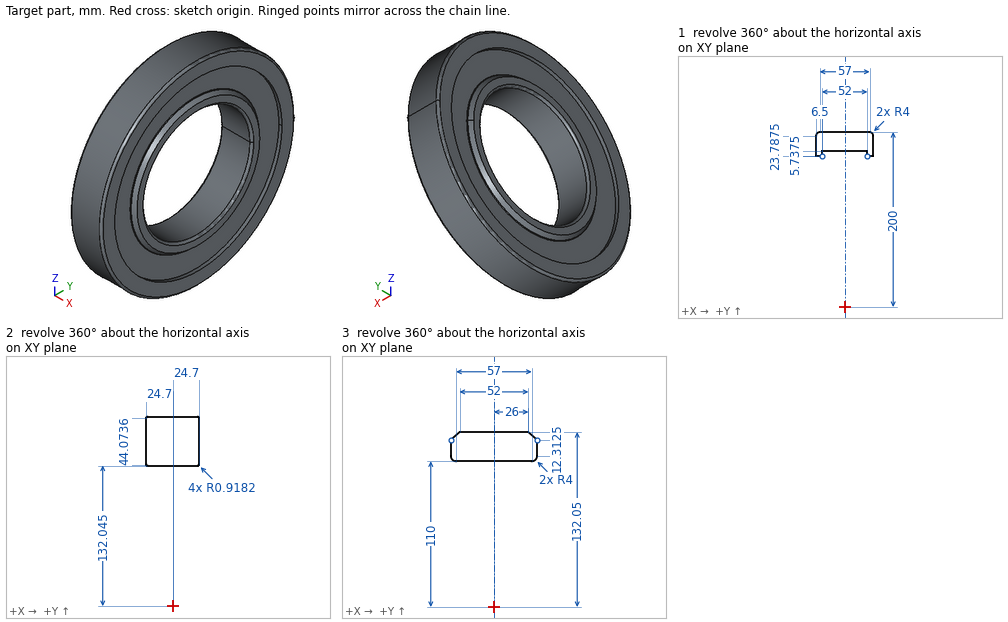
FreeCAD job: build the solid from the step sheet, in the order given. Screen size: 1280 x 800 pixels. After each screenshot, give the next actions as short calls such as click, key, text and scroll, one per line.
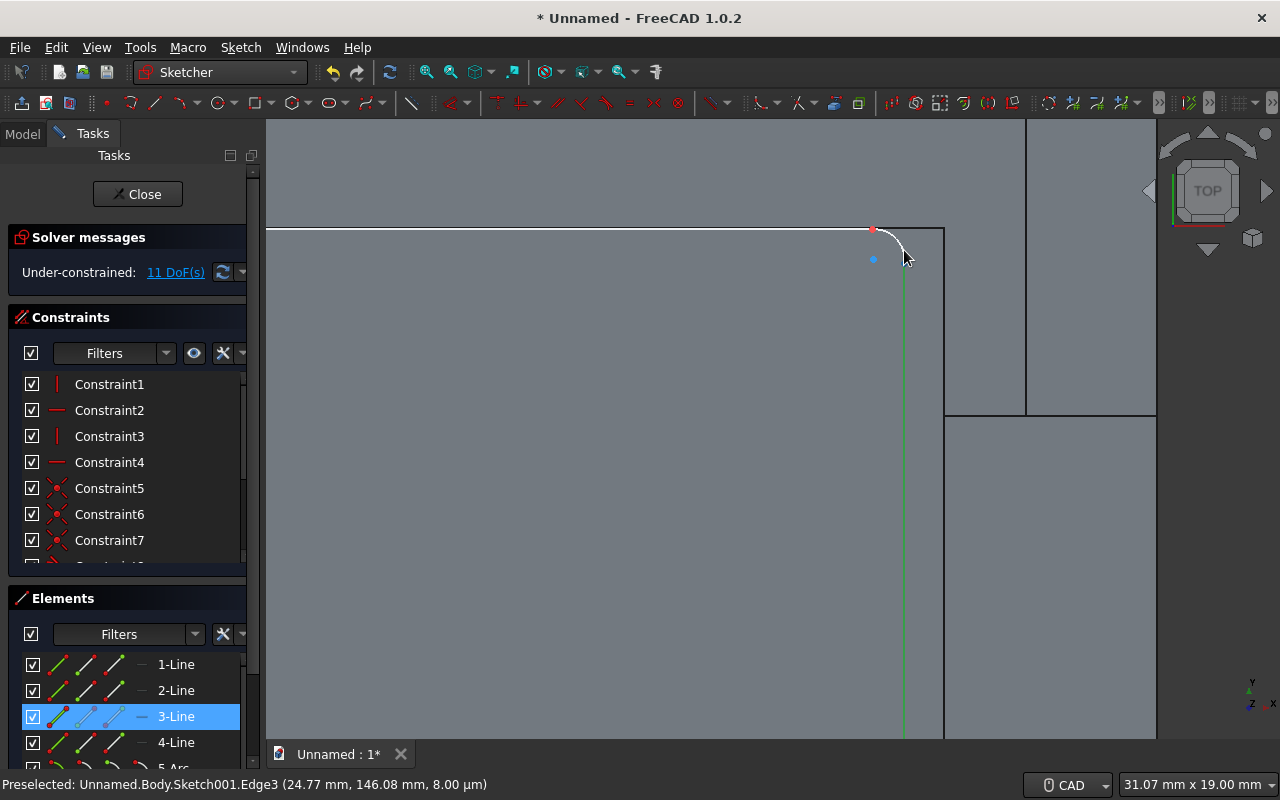
click(902, 248)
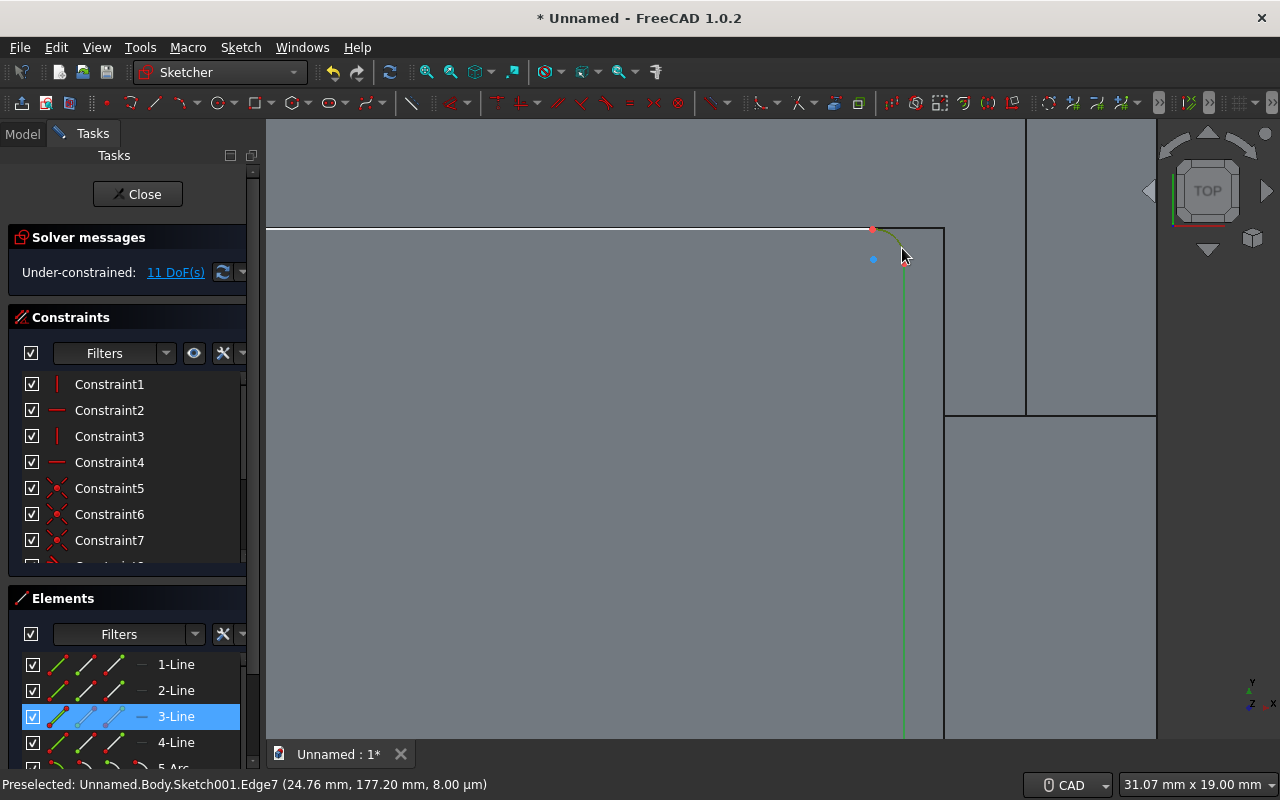
click(606, 104)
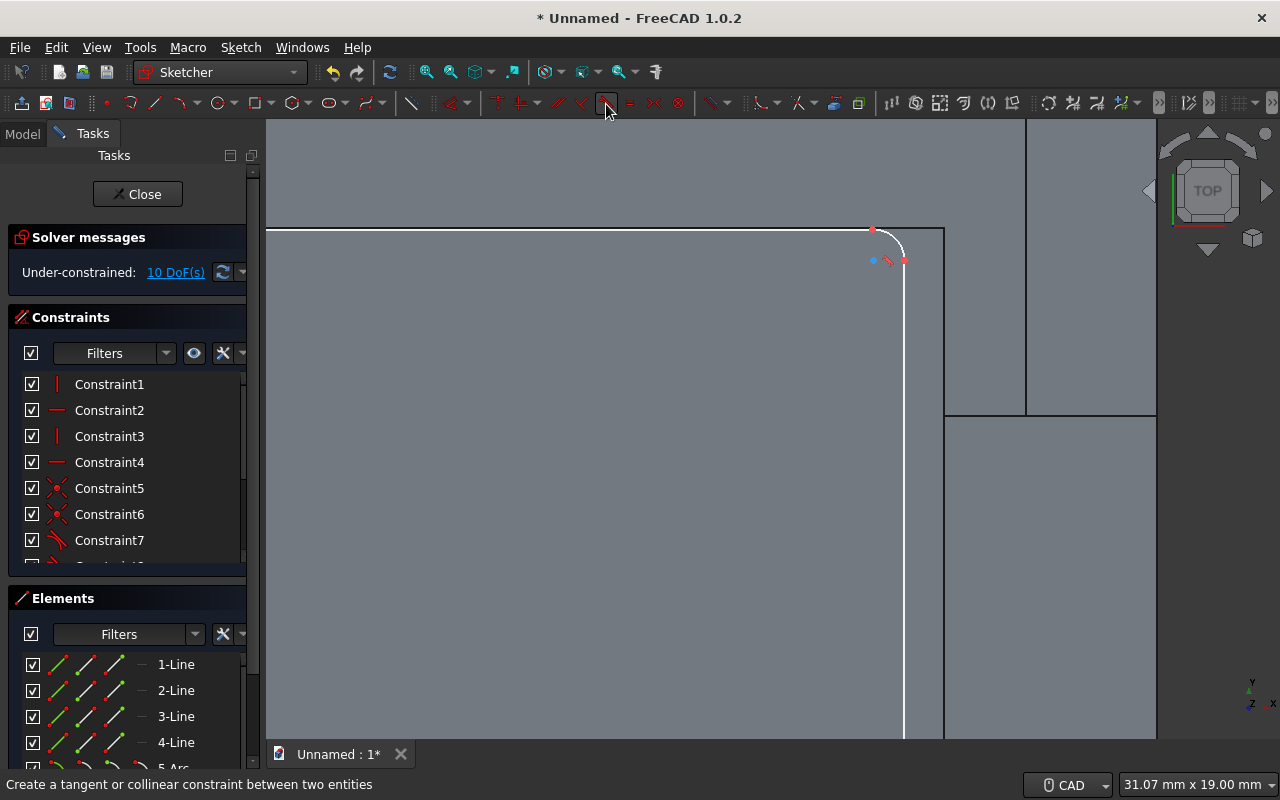
scroll(904, 250, down, 7)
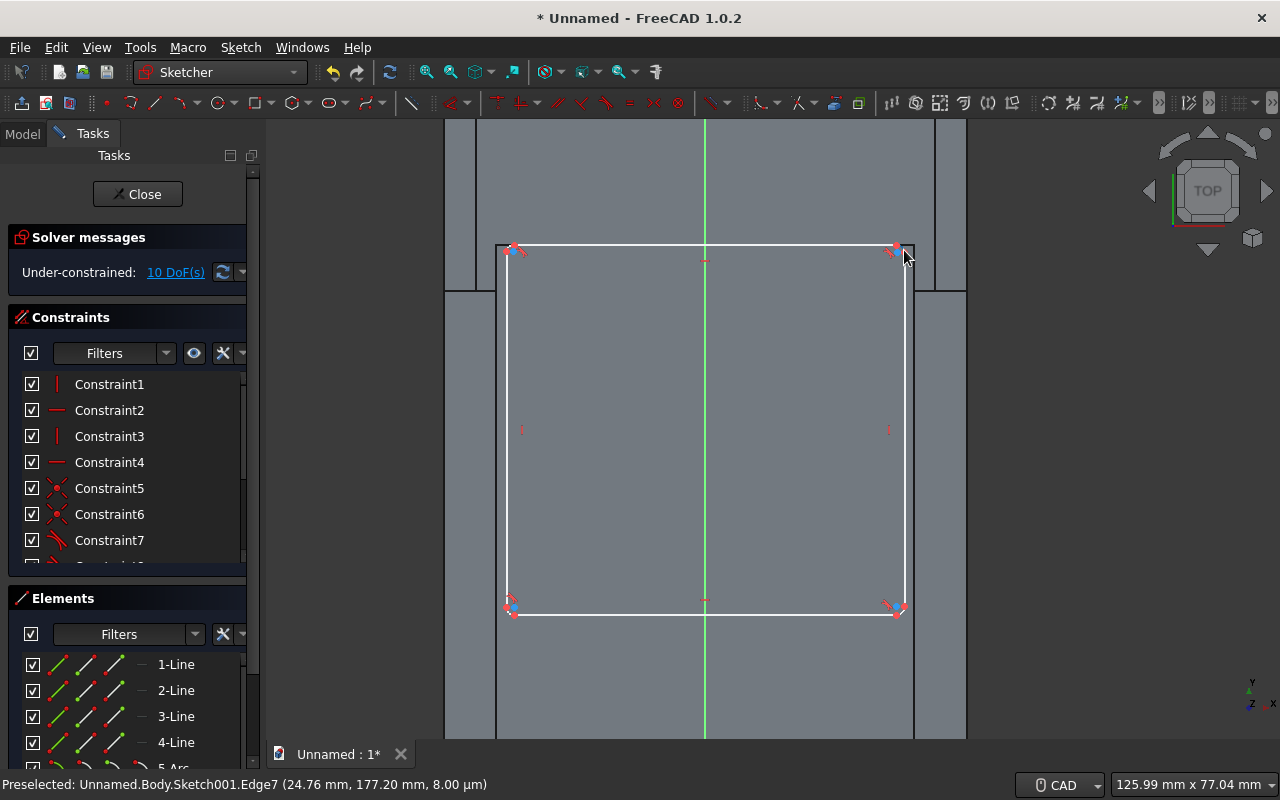
click(782, 245)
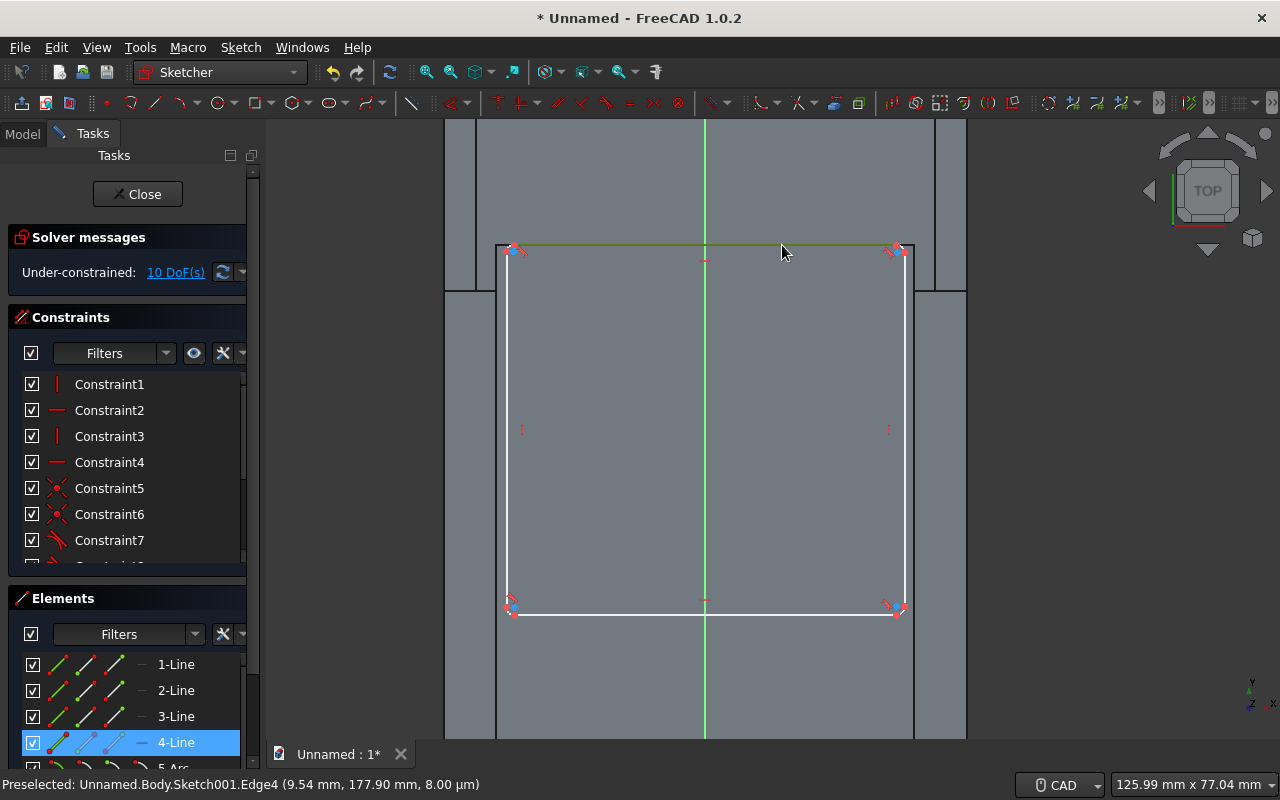
scroll(902, 247, up, 5)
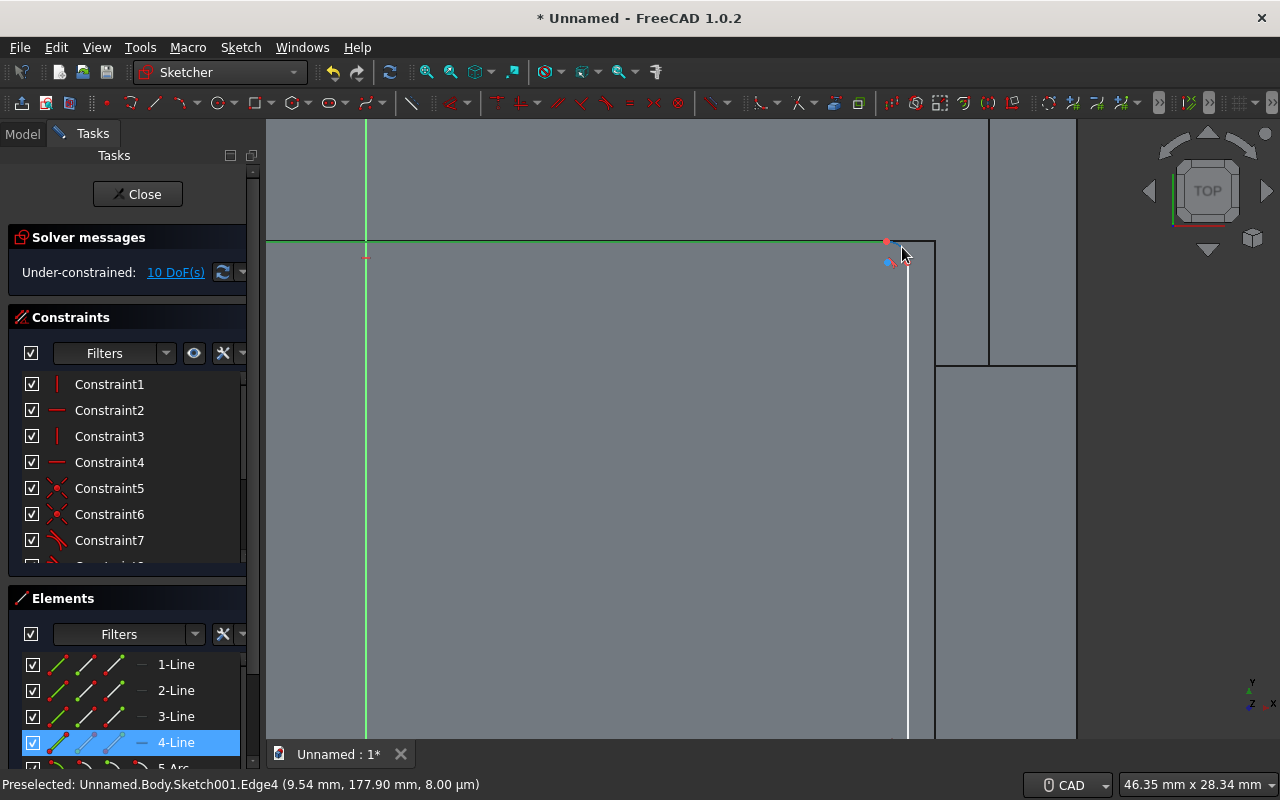
click(901, 247)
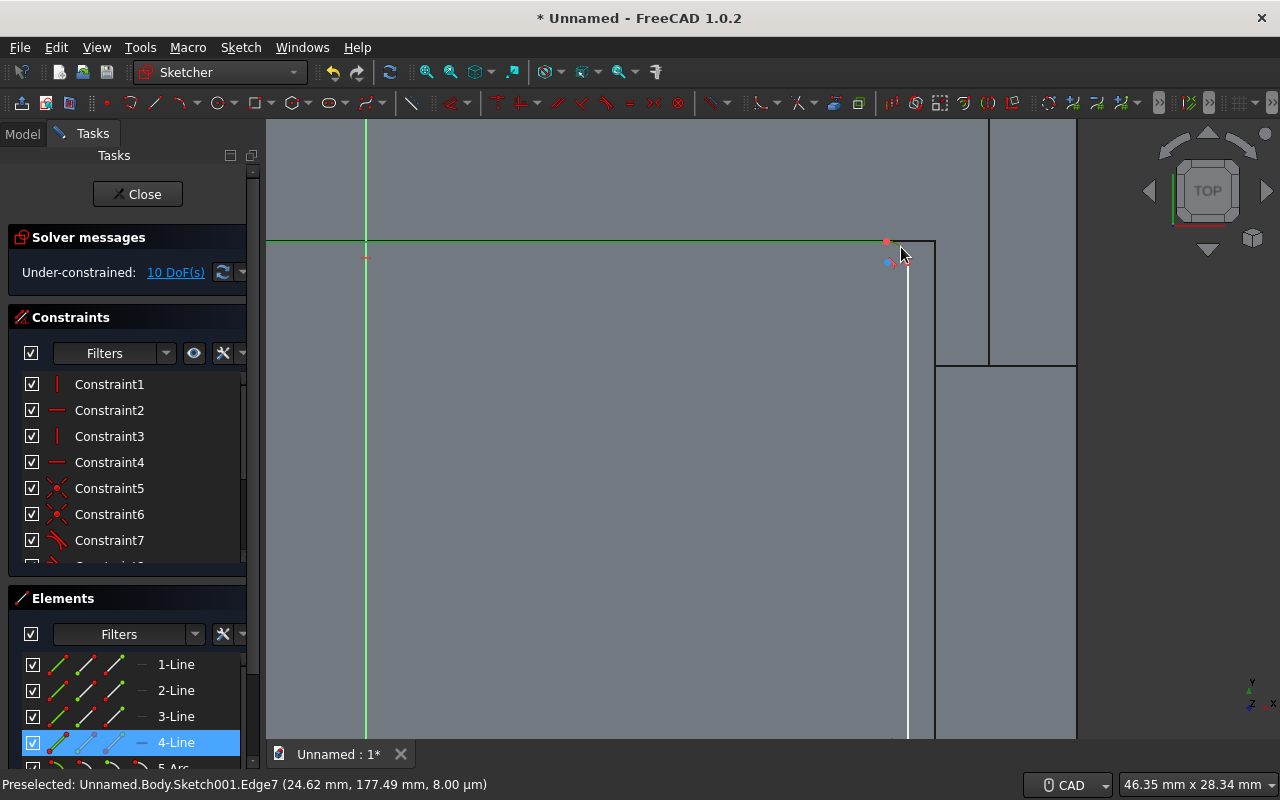
click(606, 104)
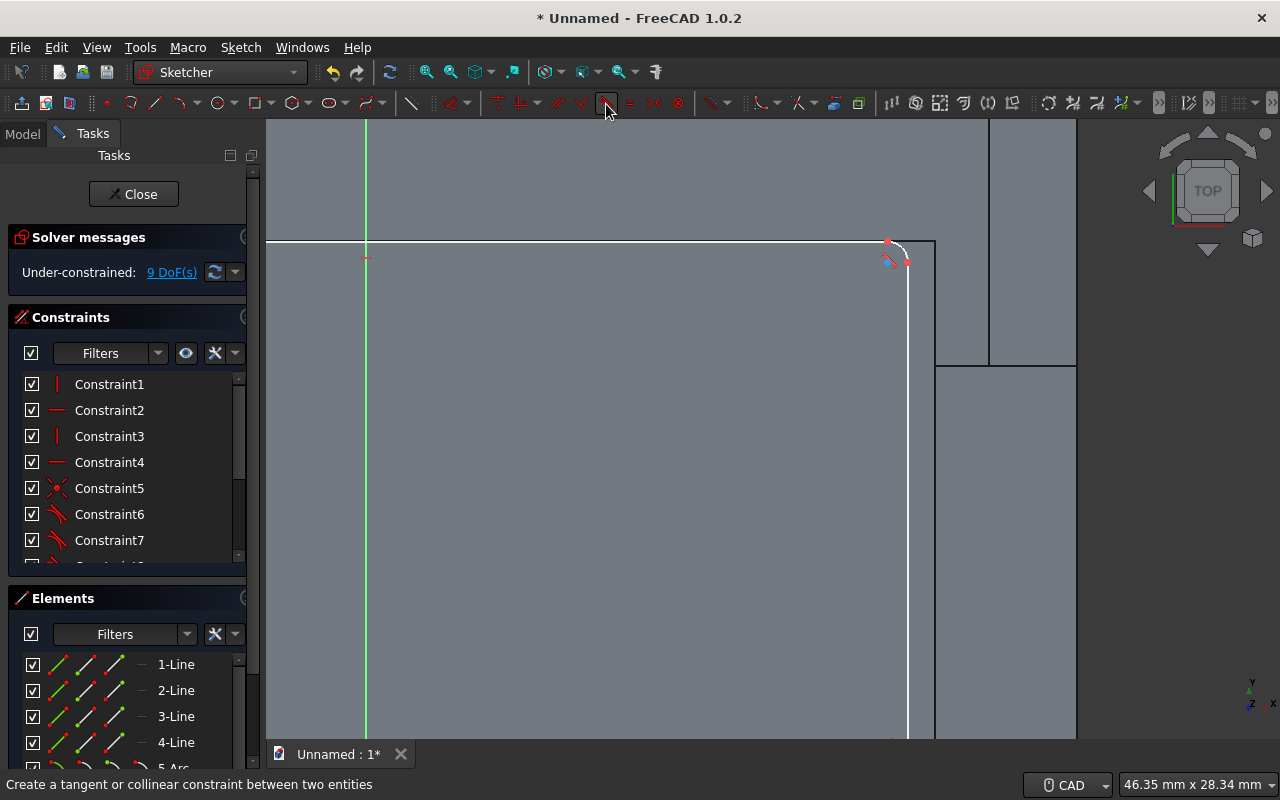
click(575, 242)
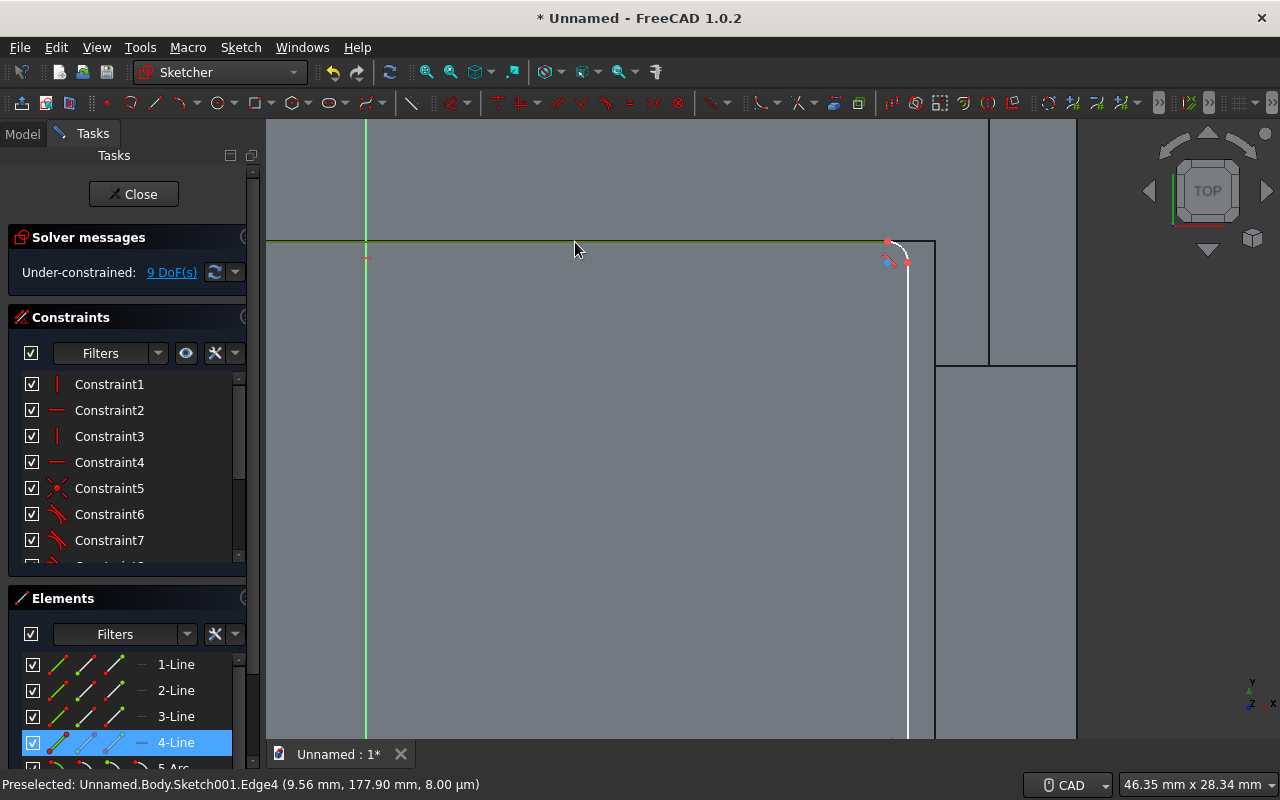
scroll(902, 246, down, 5)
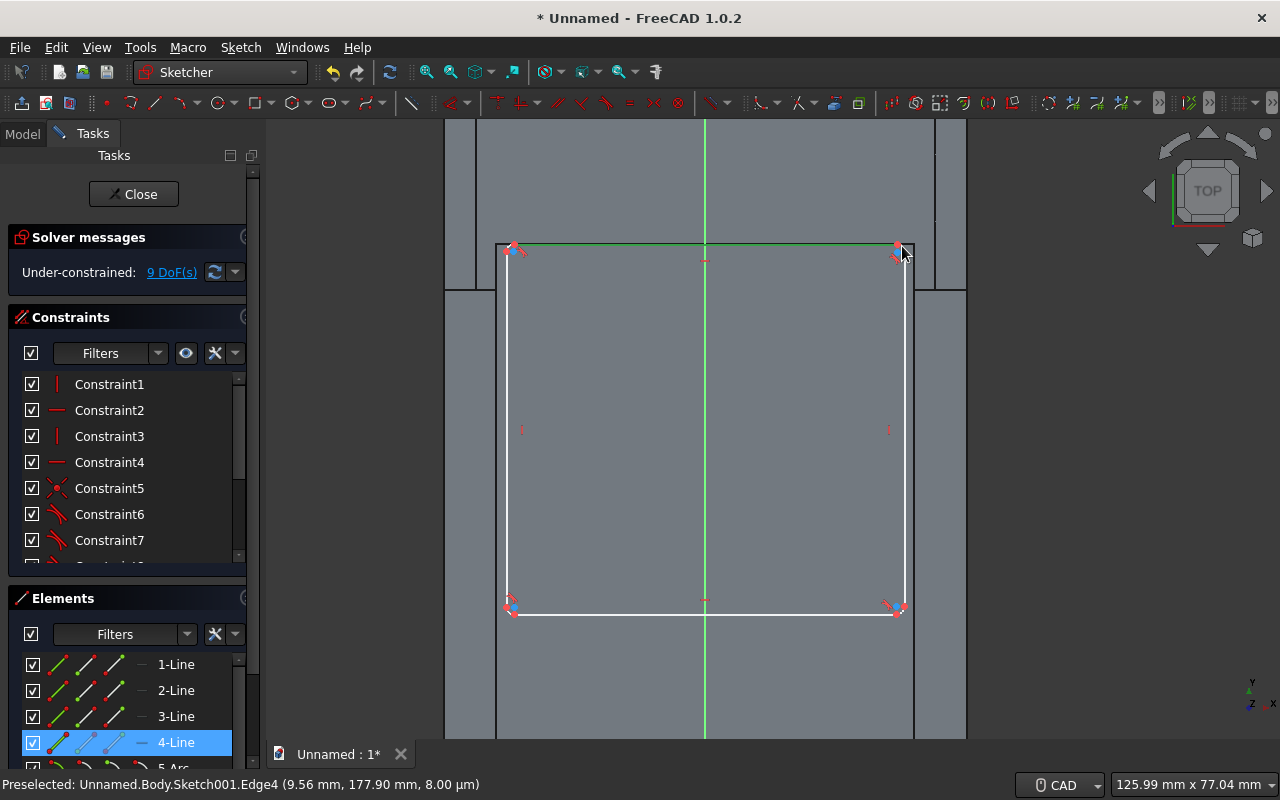
scroll(509, 246, up, 5)